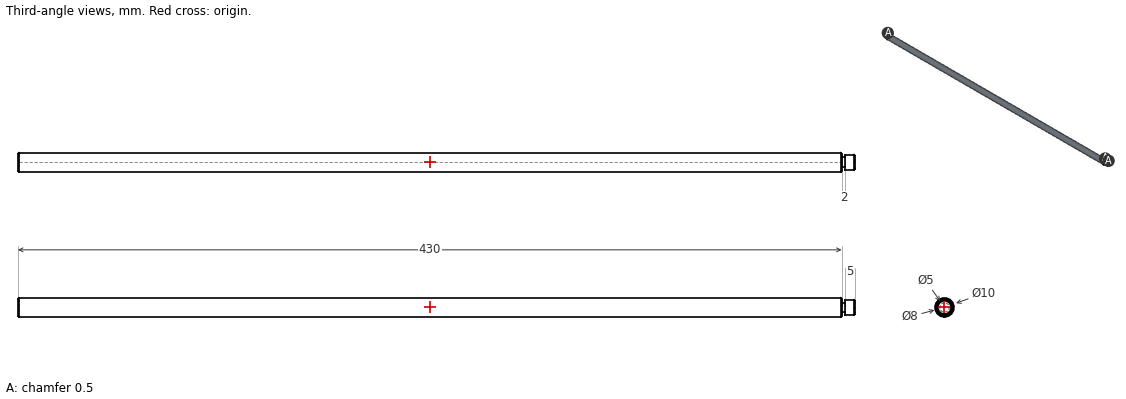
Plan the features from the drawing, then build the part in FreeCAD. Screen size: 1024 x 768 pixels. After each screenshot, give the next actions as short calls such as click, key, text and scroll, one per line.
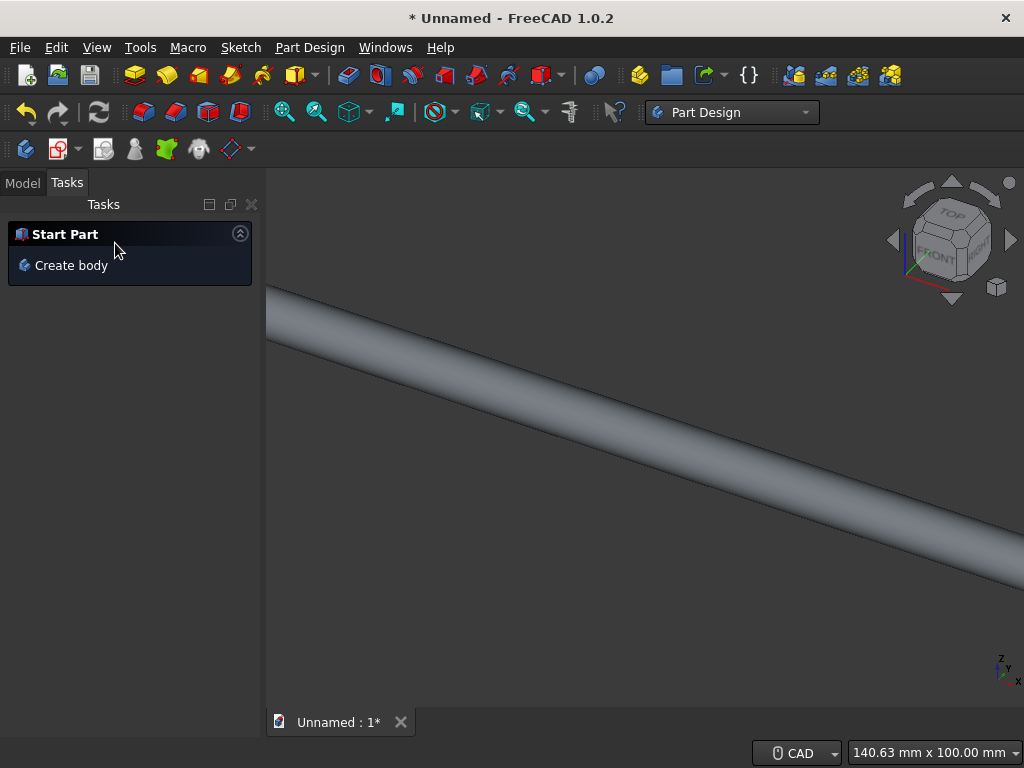
click(286, 112)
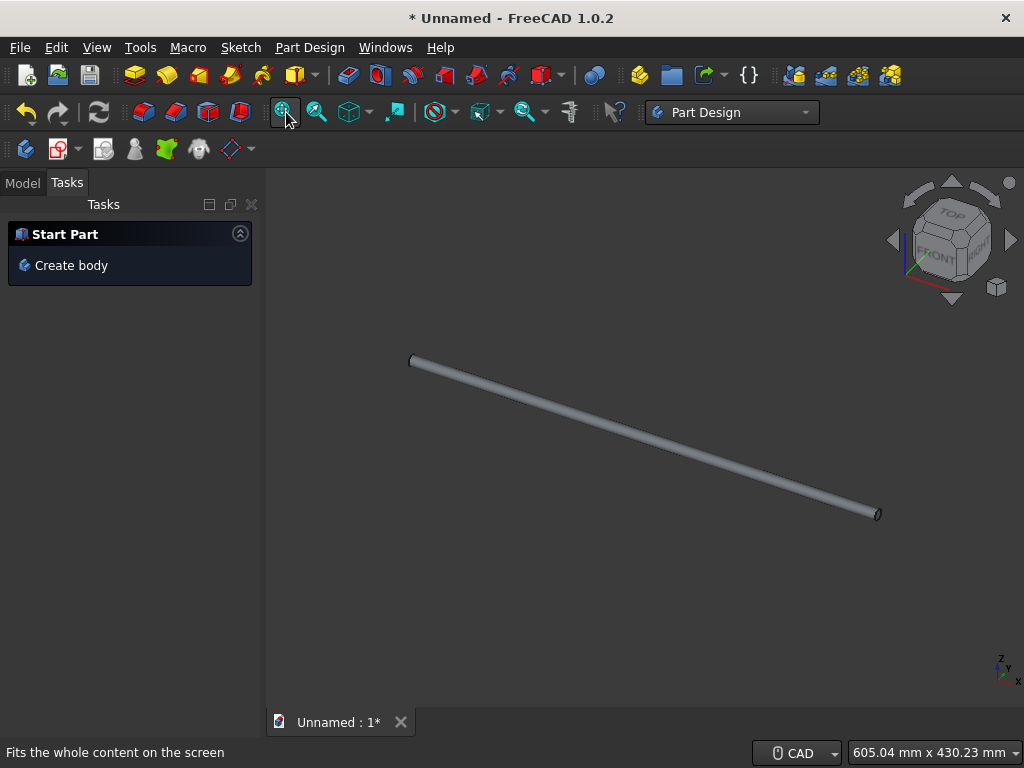
key(0)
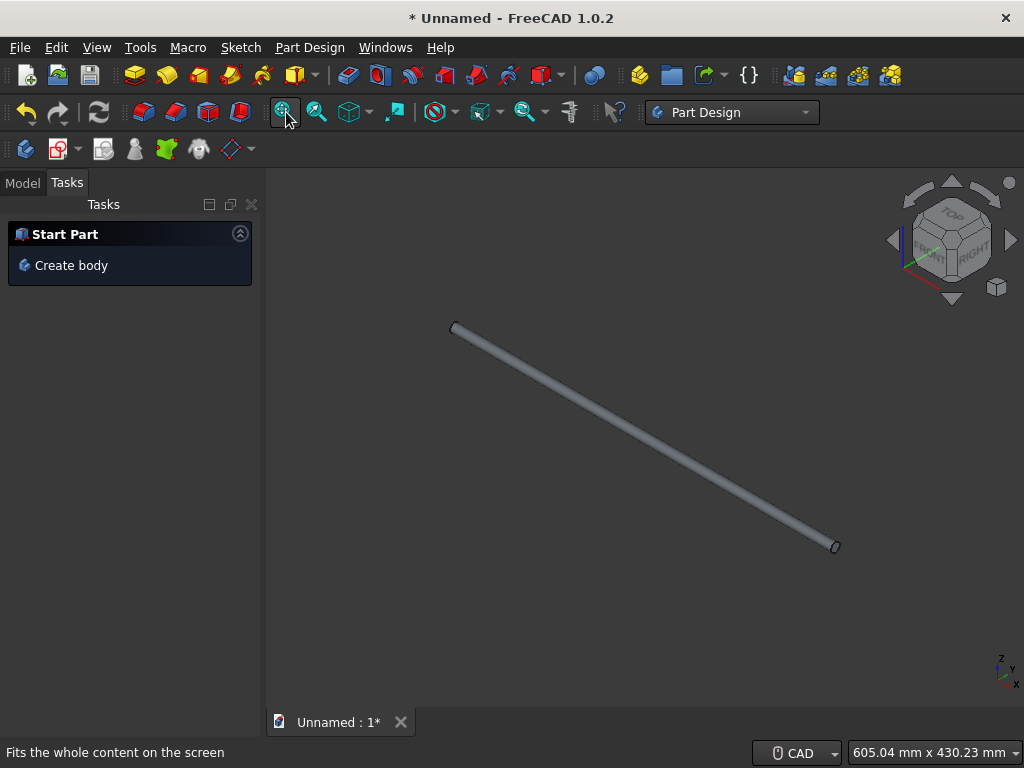
scroll(835, 546, up, 4)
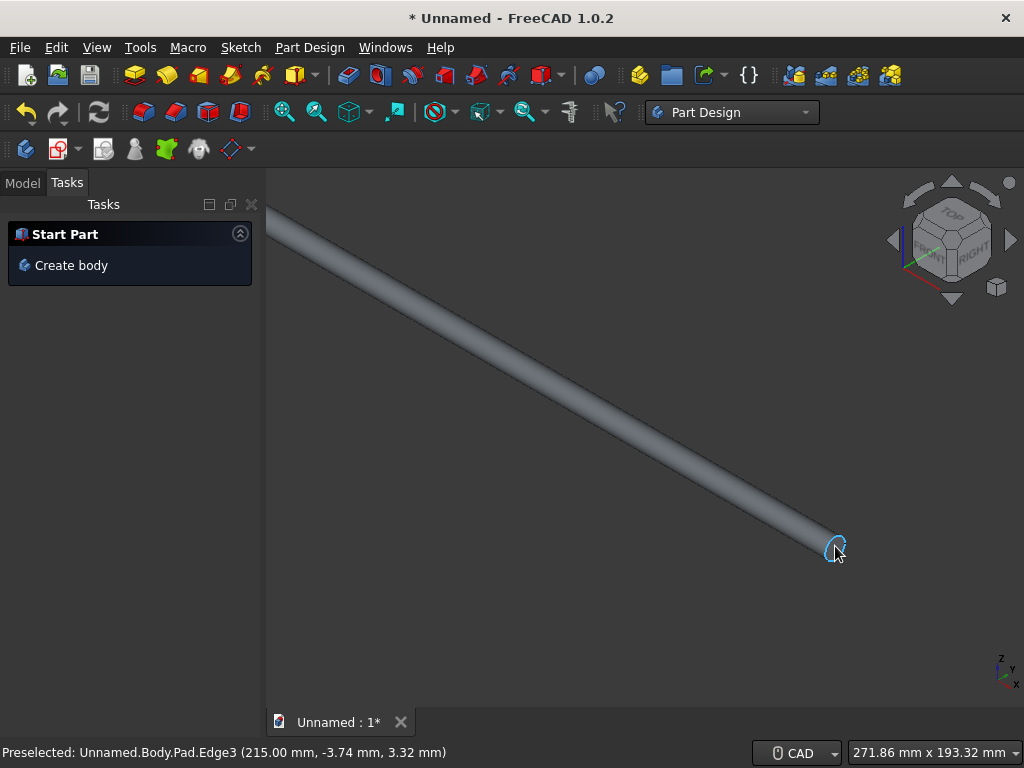
click(838, 546)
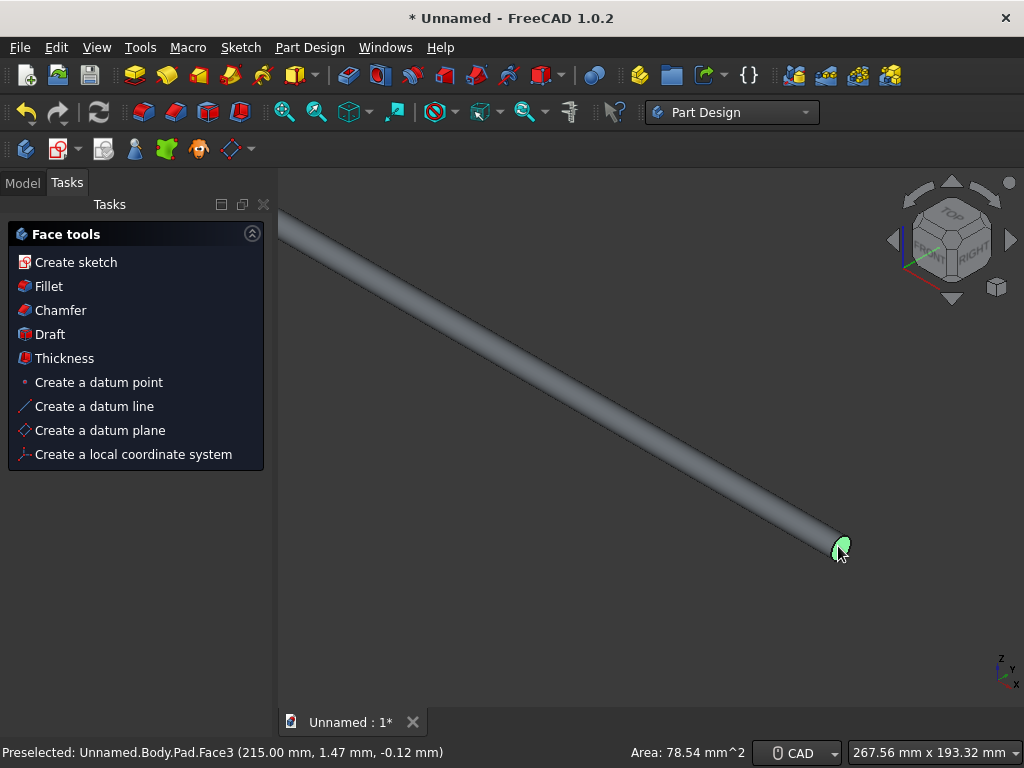
click(58, 150)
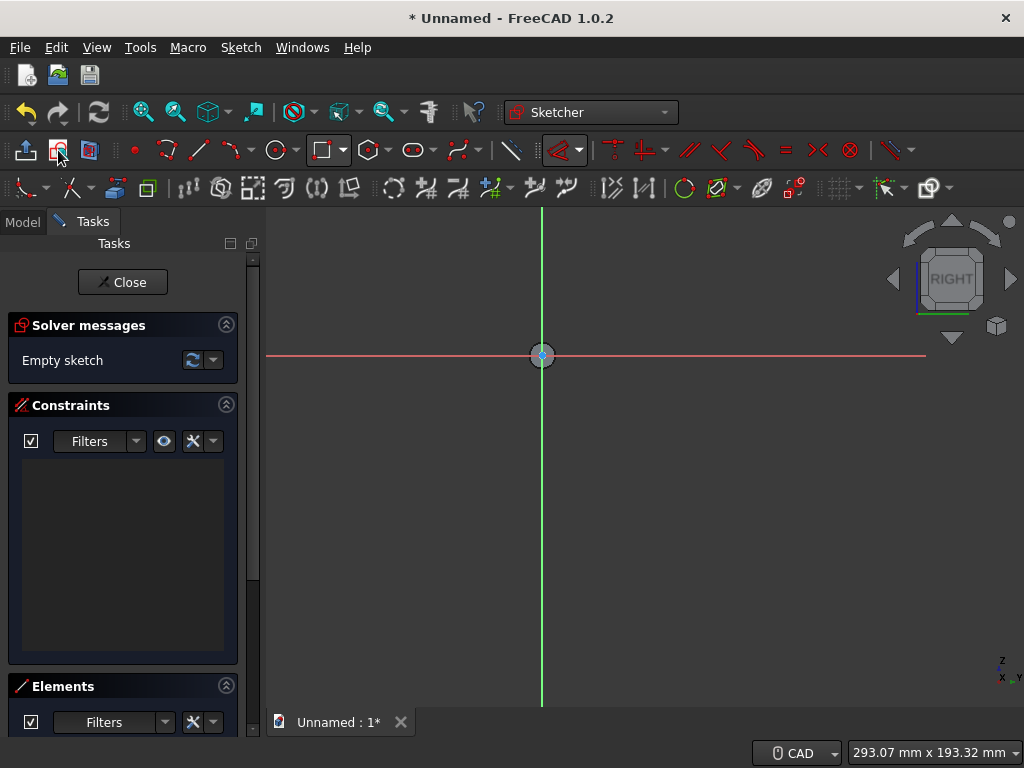
scroll(541, 350, up, 15)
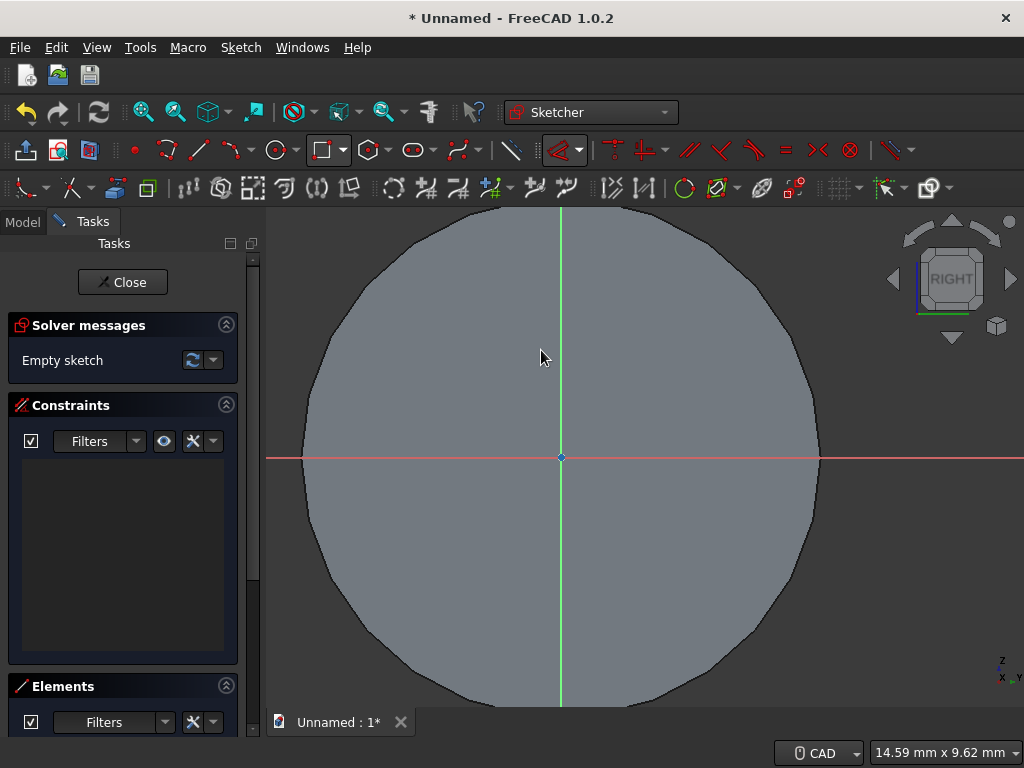
click(276, 150)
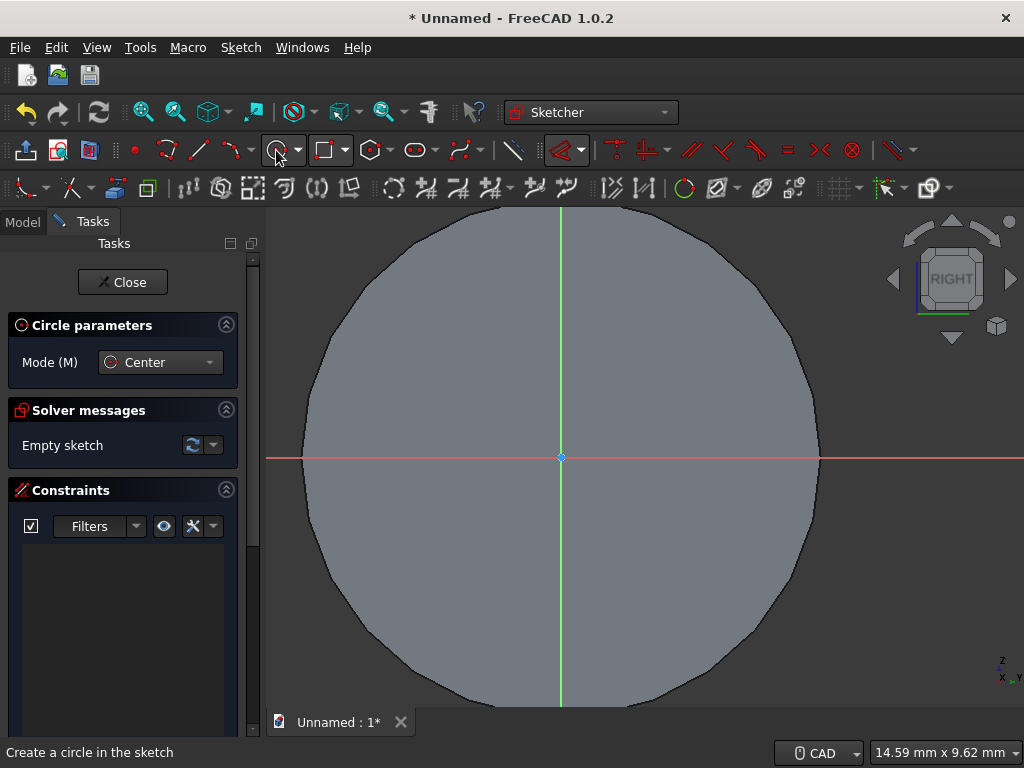
click(561, 458)
move(653, 366)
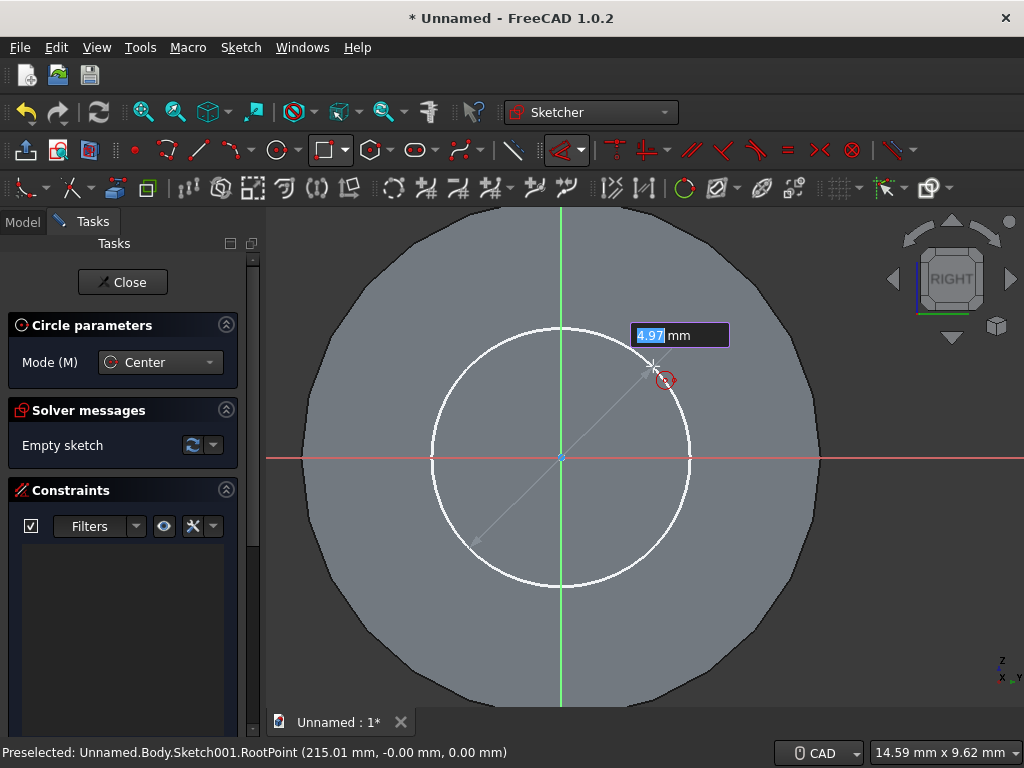
text(5)
key(Return)
key(Escape)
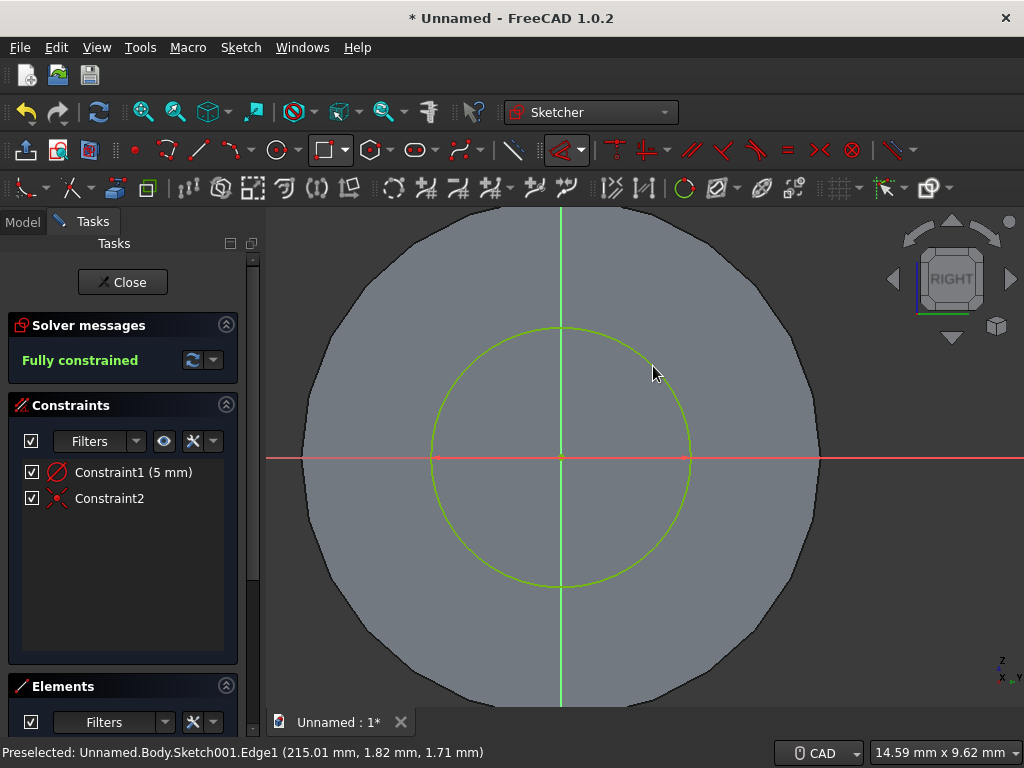
click(123, 282)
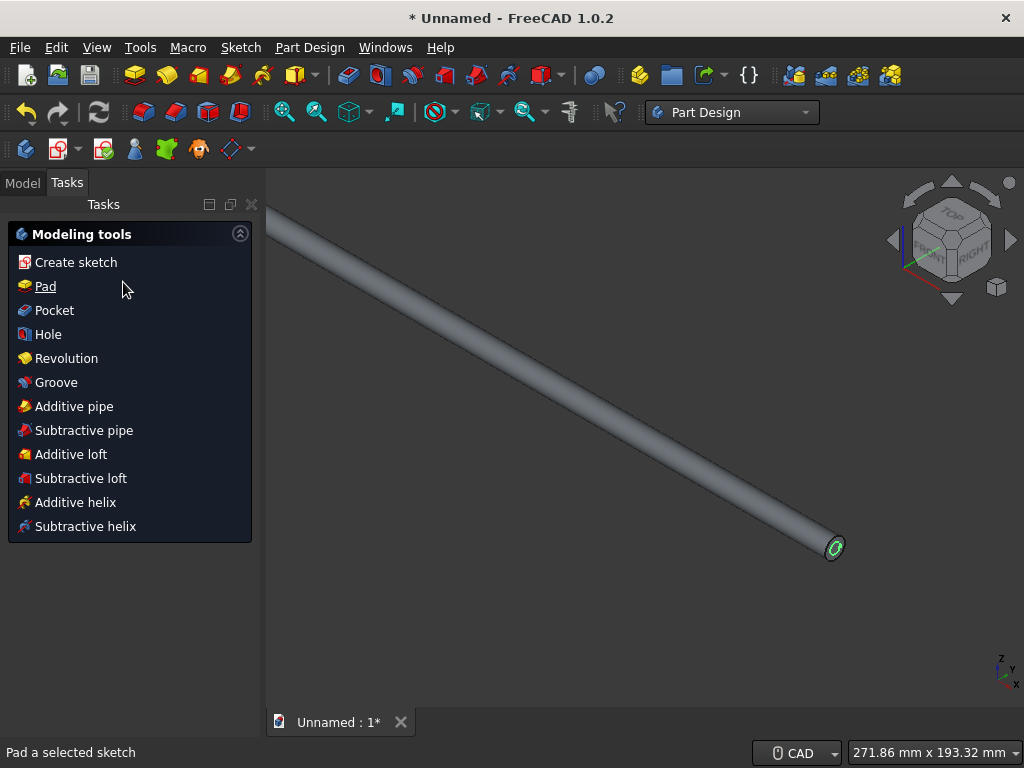
click(136, 76)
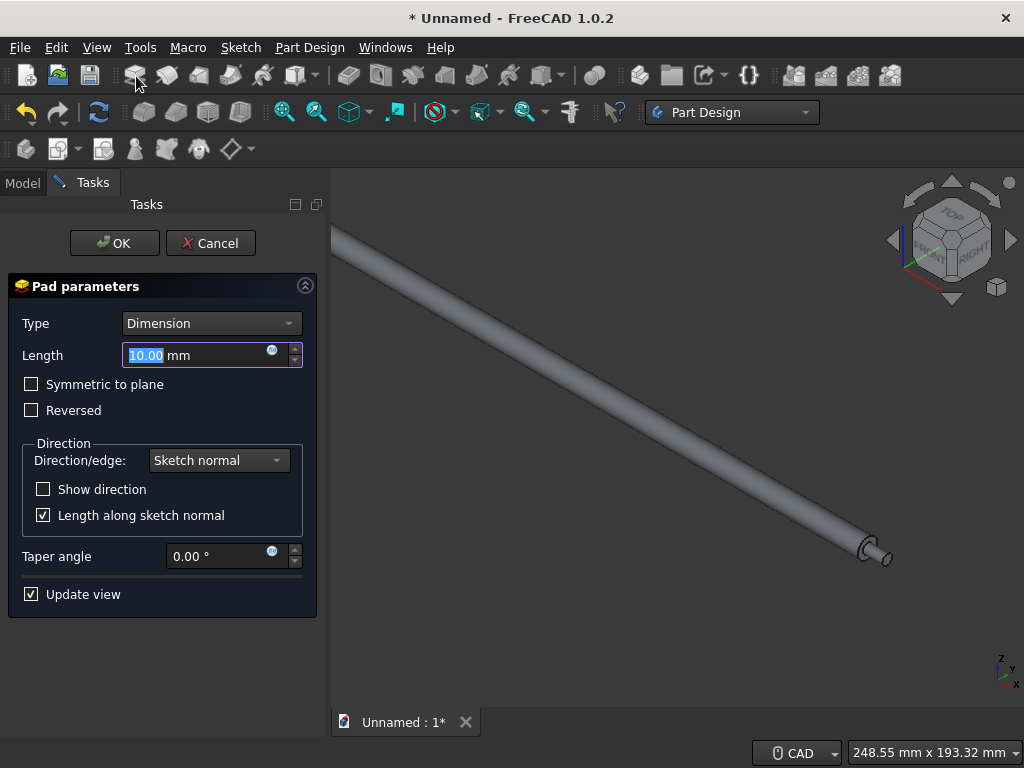
text(2)
key(Tab)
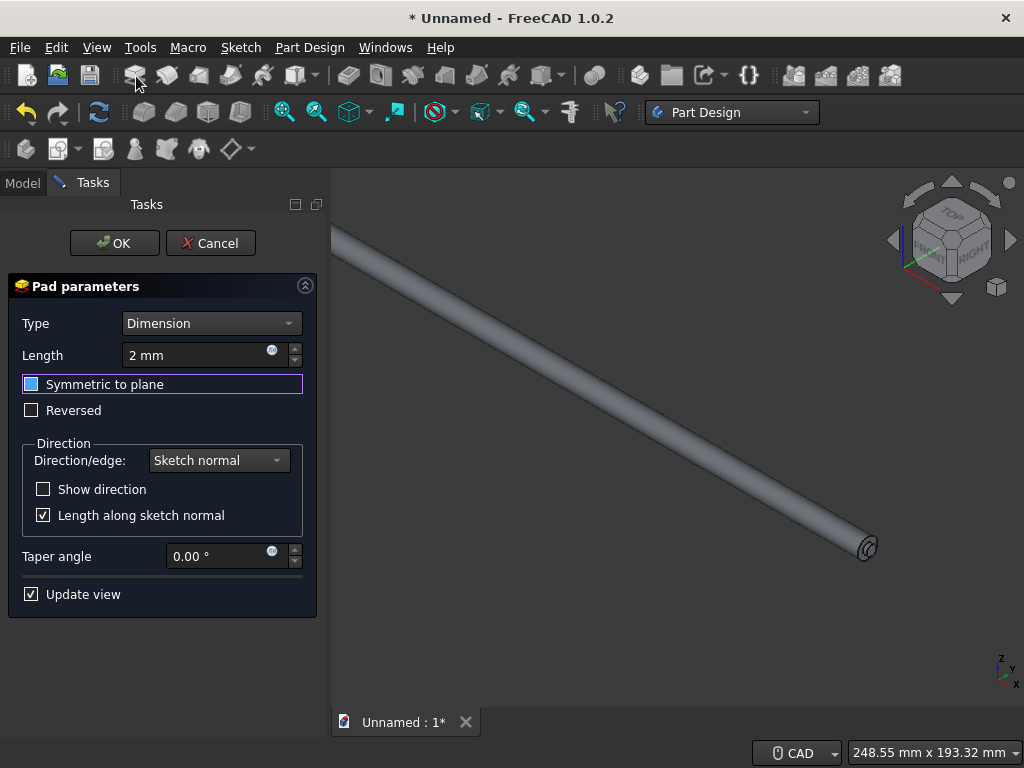
click(115, 243)